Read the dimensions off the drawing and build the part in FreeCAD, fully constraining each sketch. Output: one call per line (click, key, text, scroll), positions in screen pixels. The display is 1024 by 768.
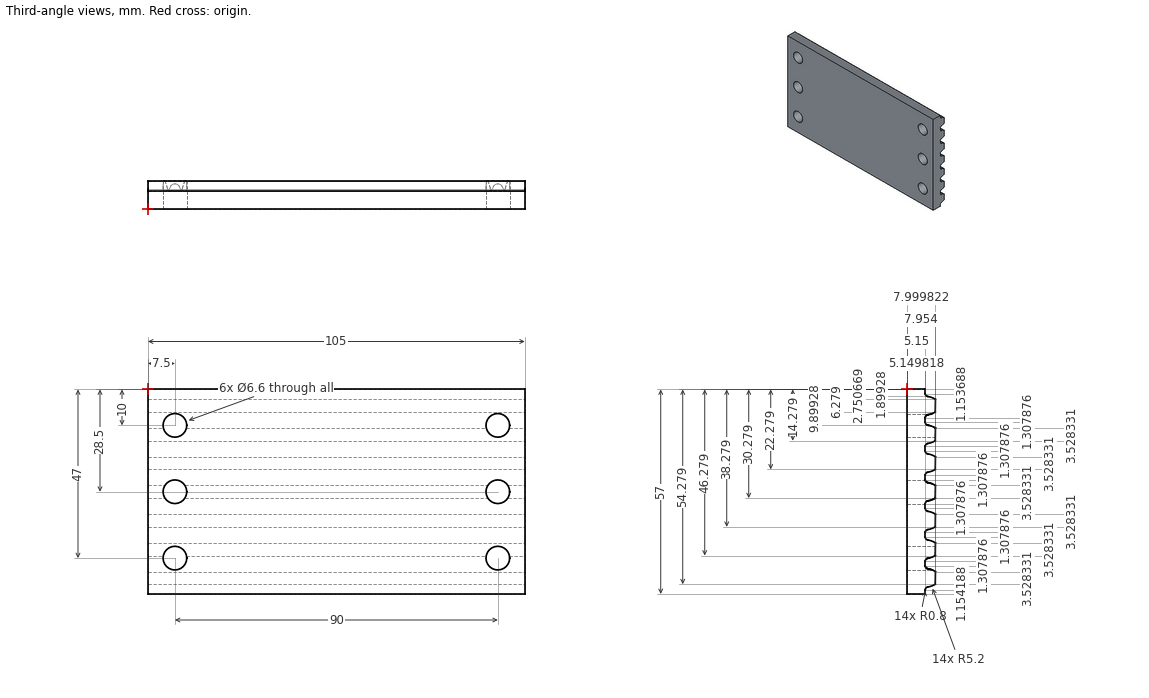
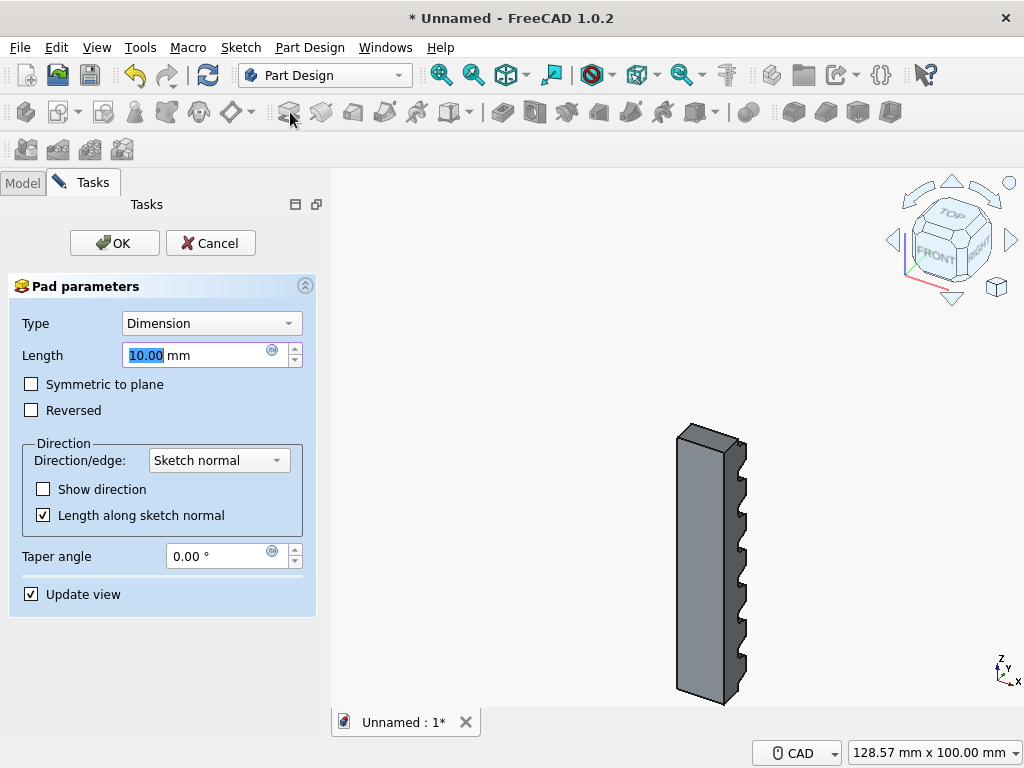
text(105)
key(Tab)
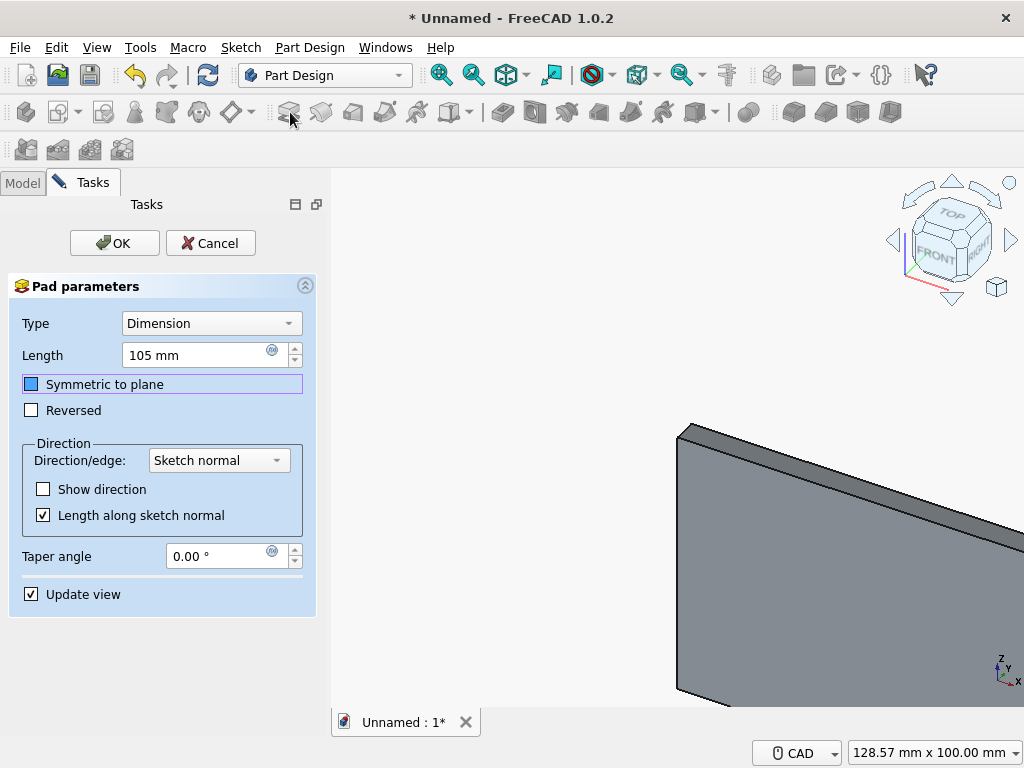
click(115, 243)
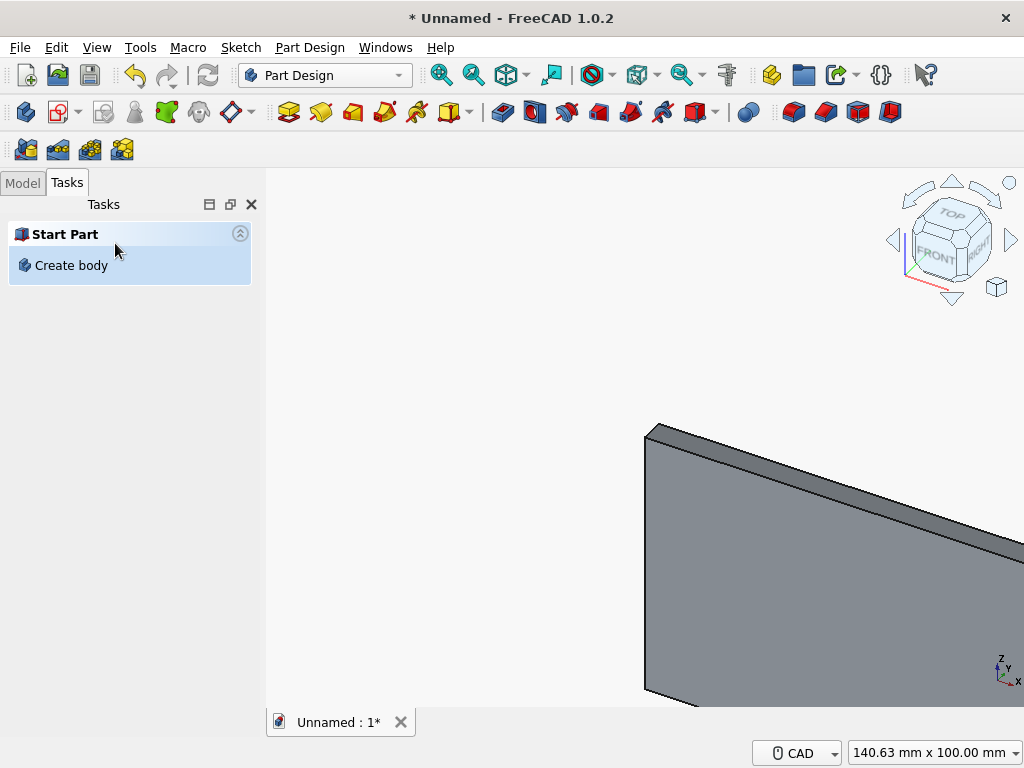
click(442, 76)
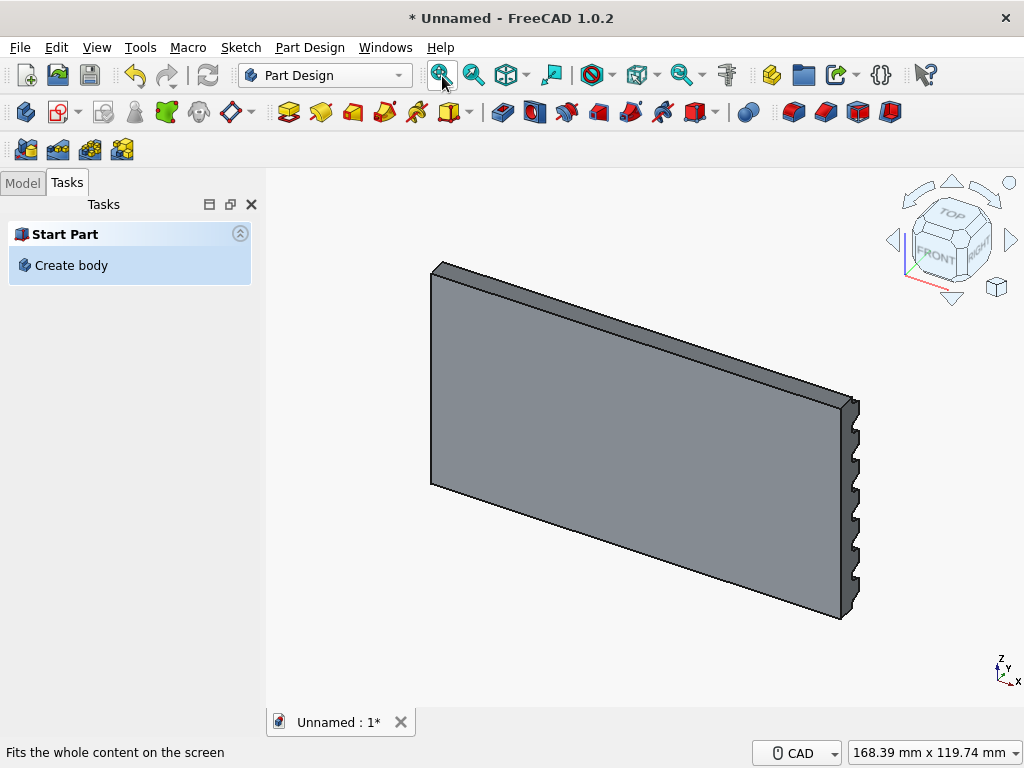
click(636, 445)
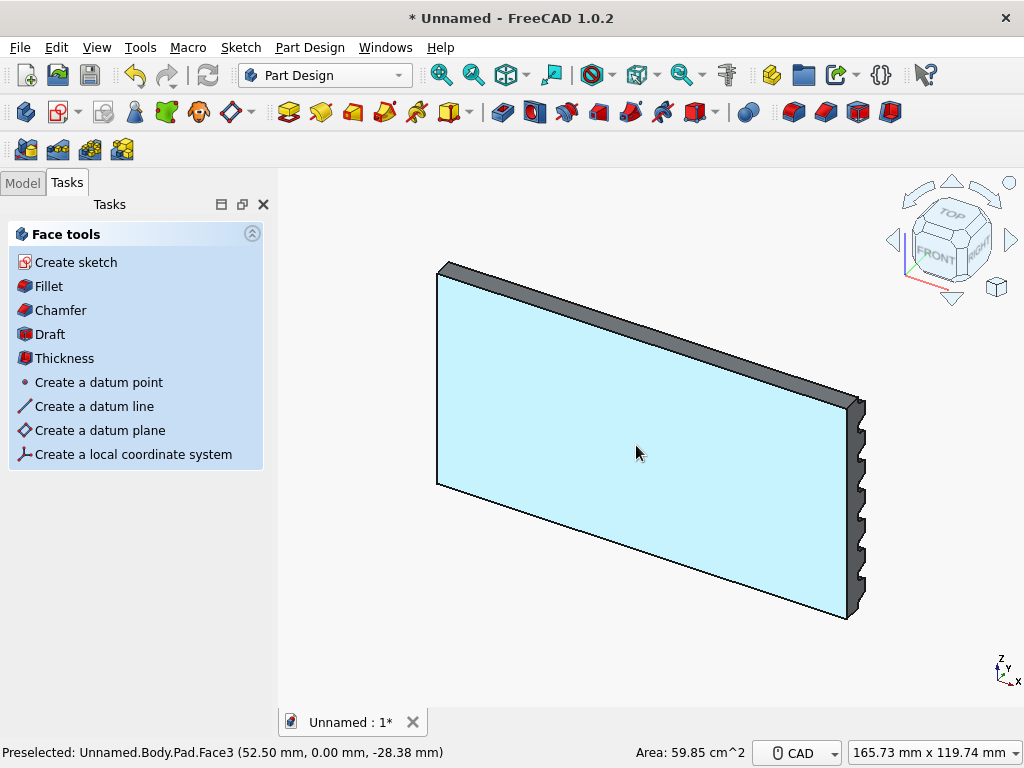
click(58, 112)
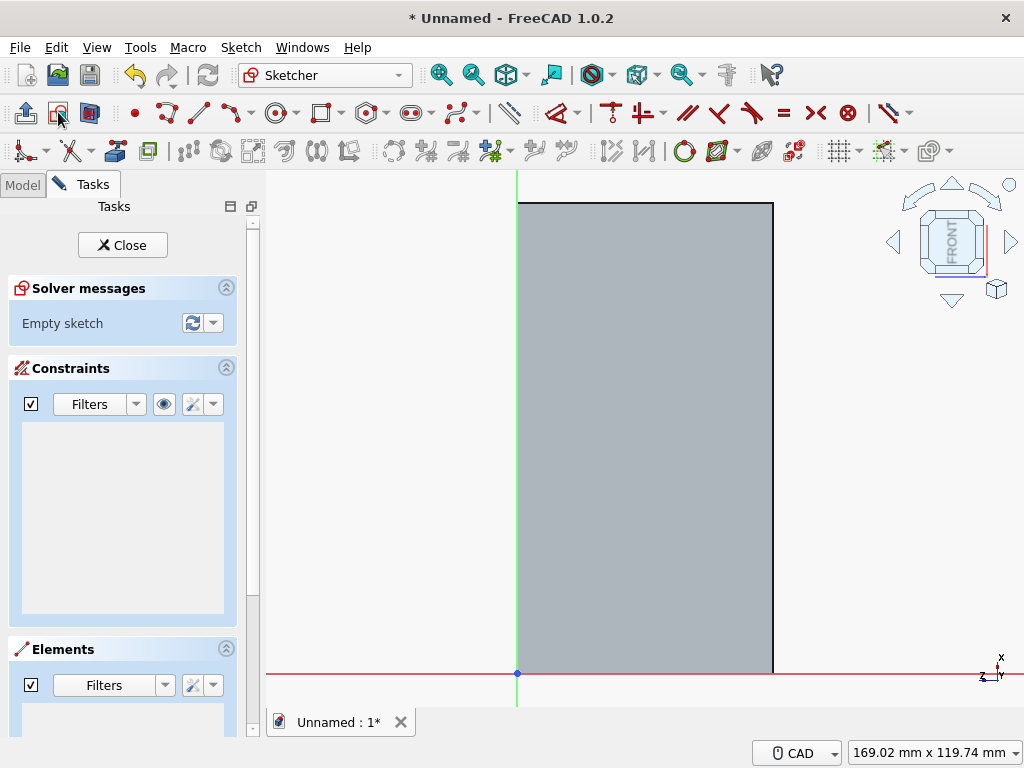
scroll(335, 396, down, 1)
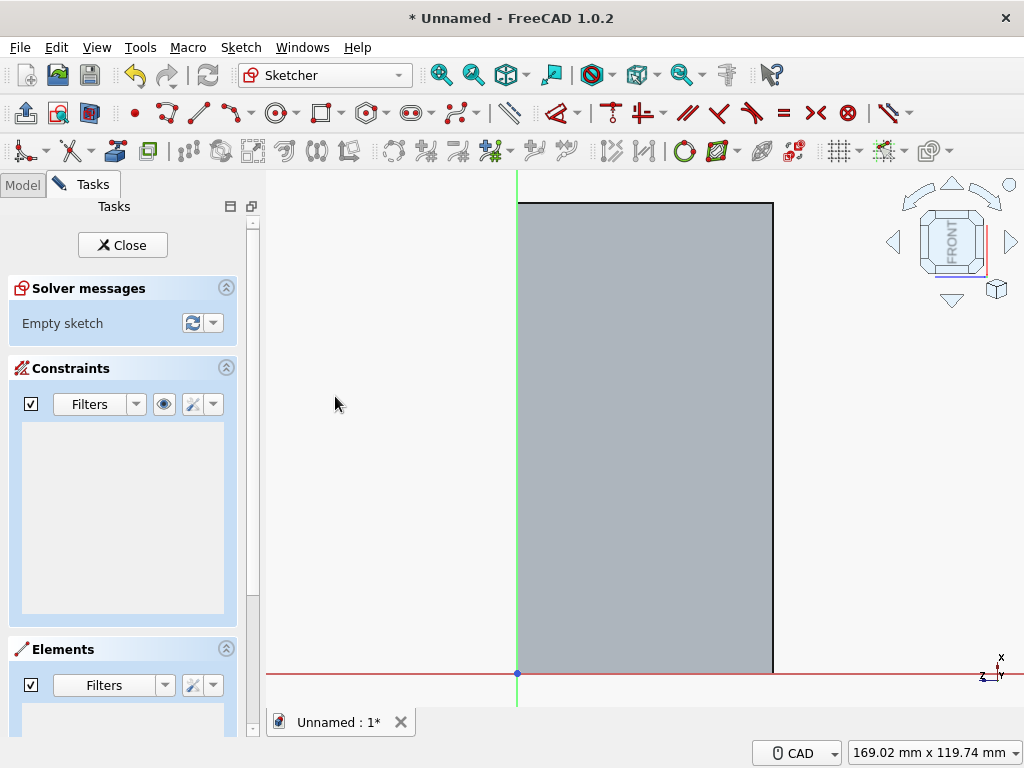
click(276, 114)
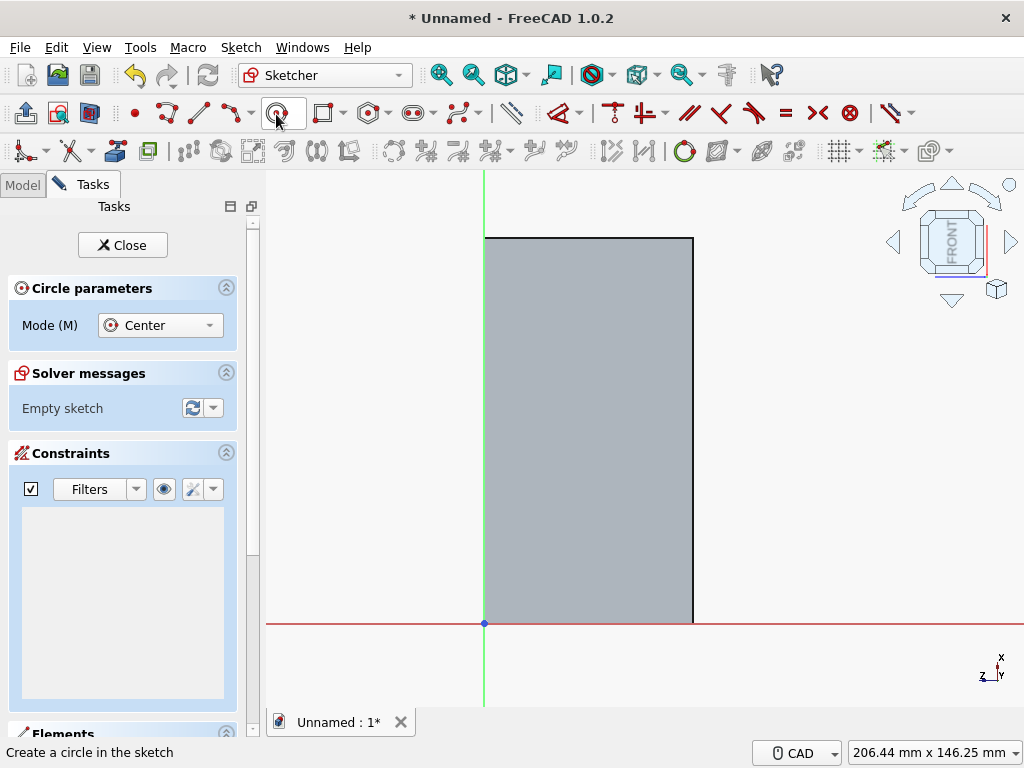
scroll(521, 596, up, 4)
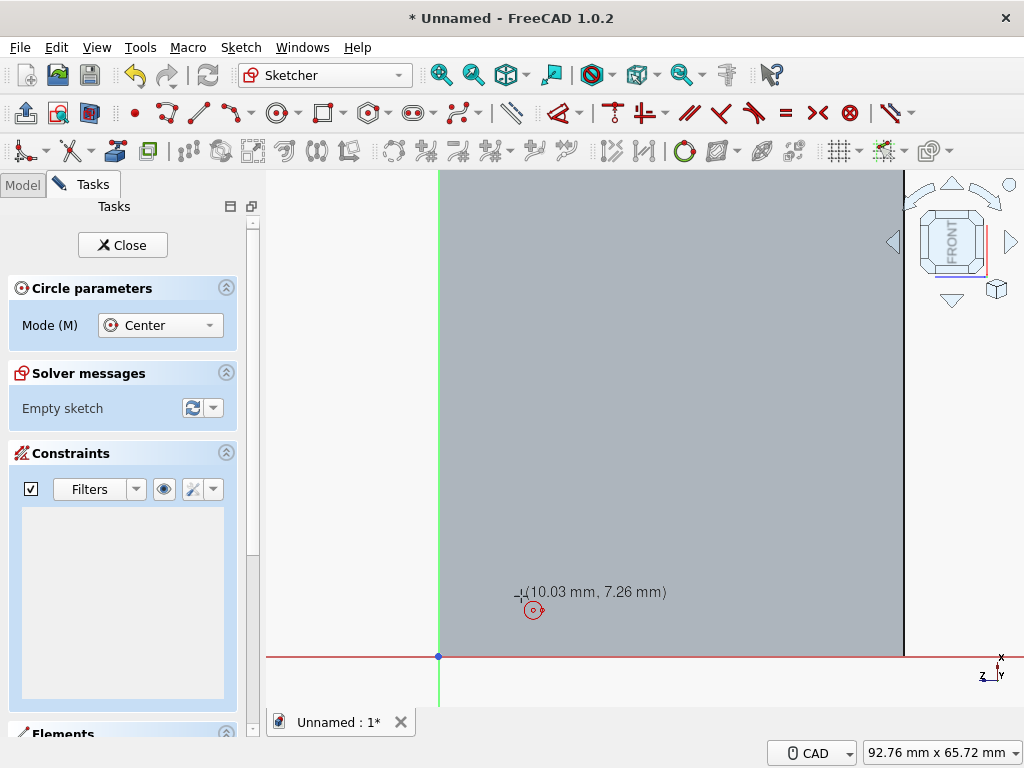
click(520, 595)
click(539, 576)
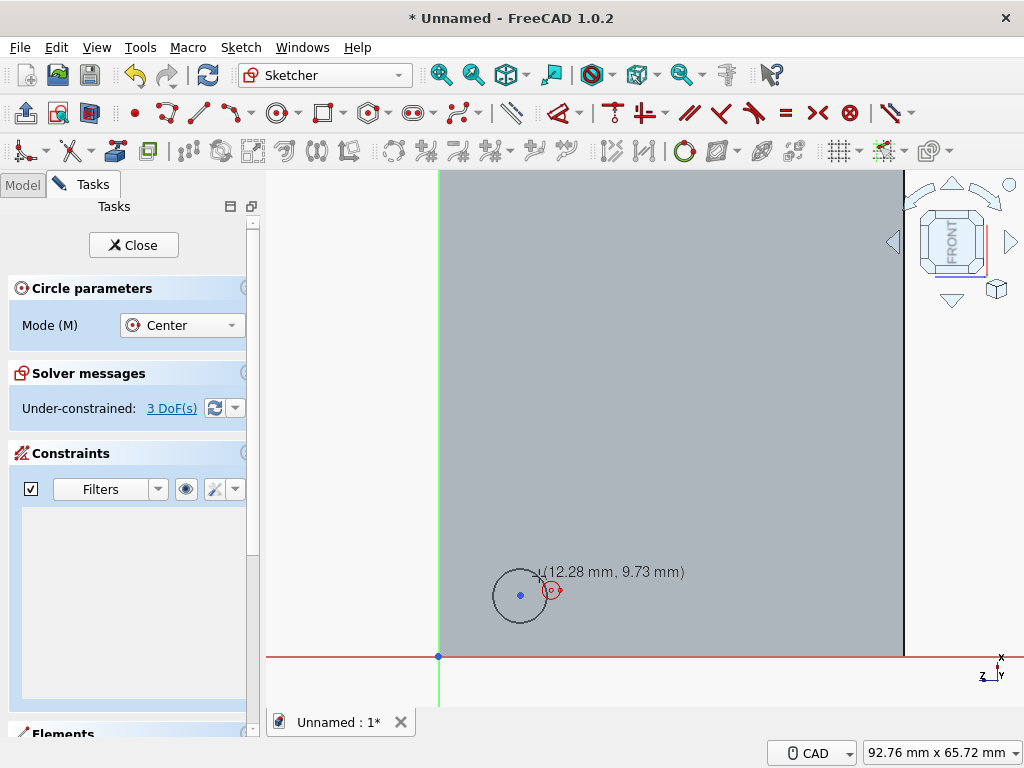
click(823, 595)
click(842, 576)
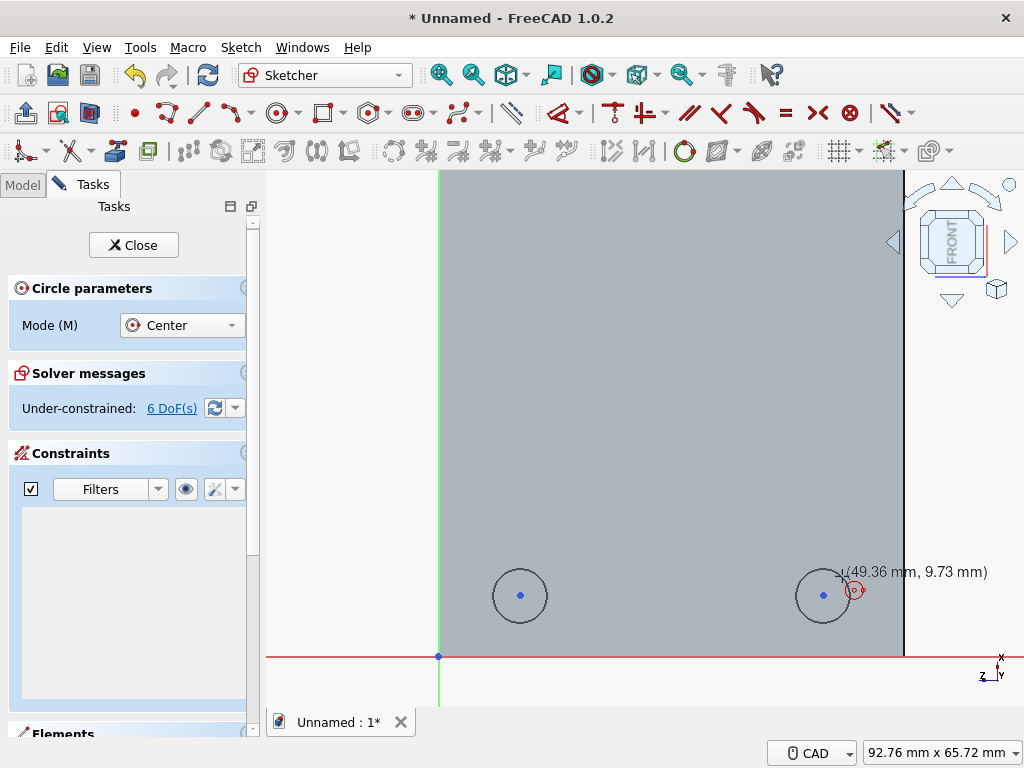
scroll(521, 597, down, 4)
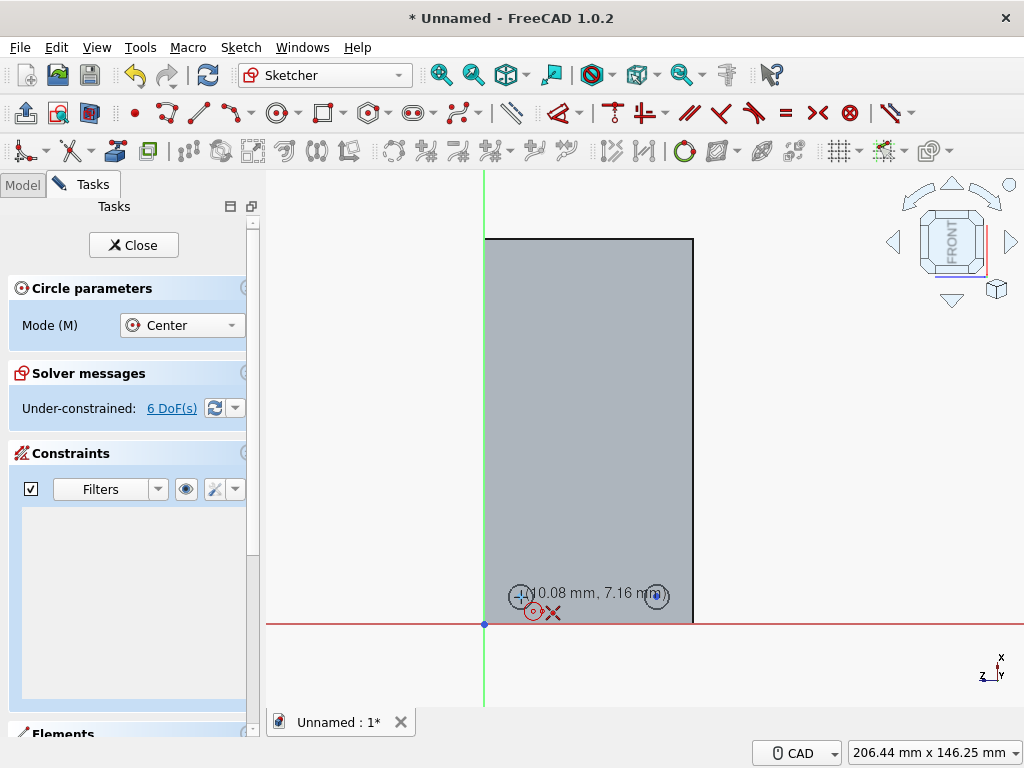
scroll(657, 266, up, 4)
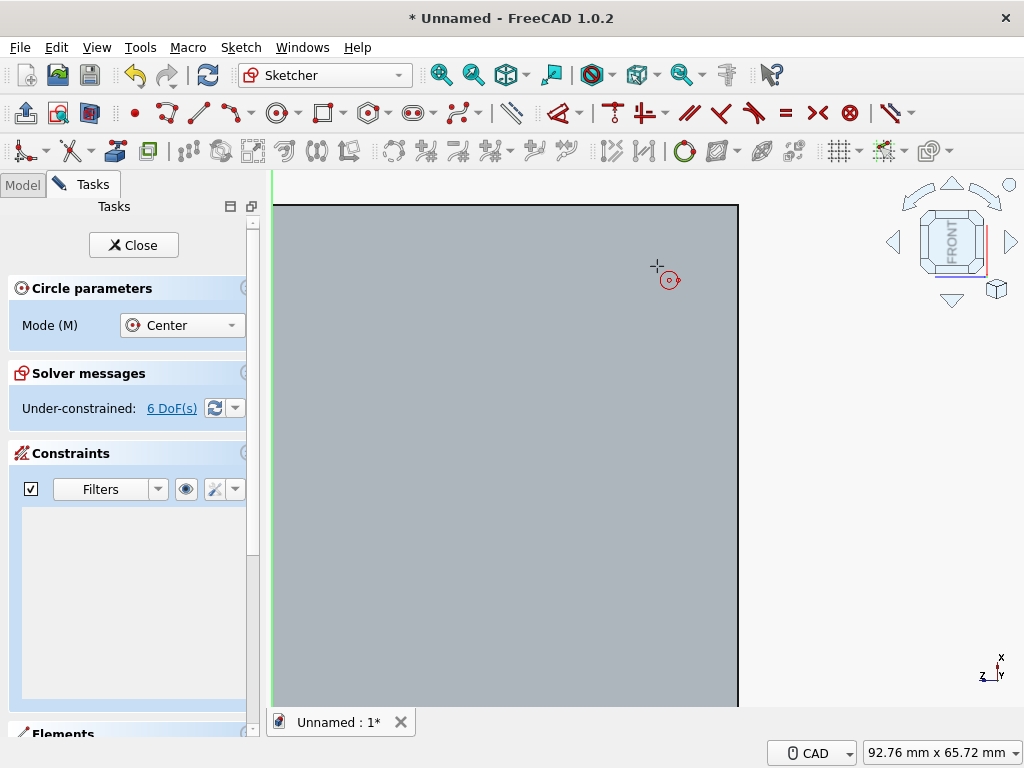
click(656, 266)
click(675, 247)